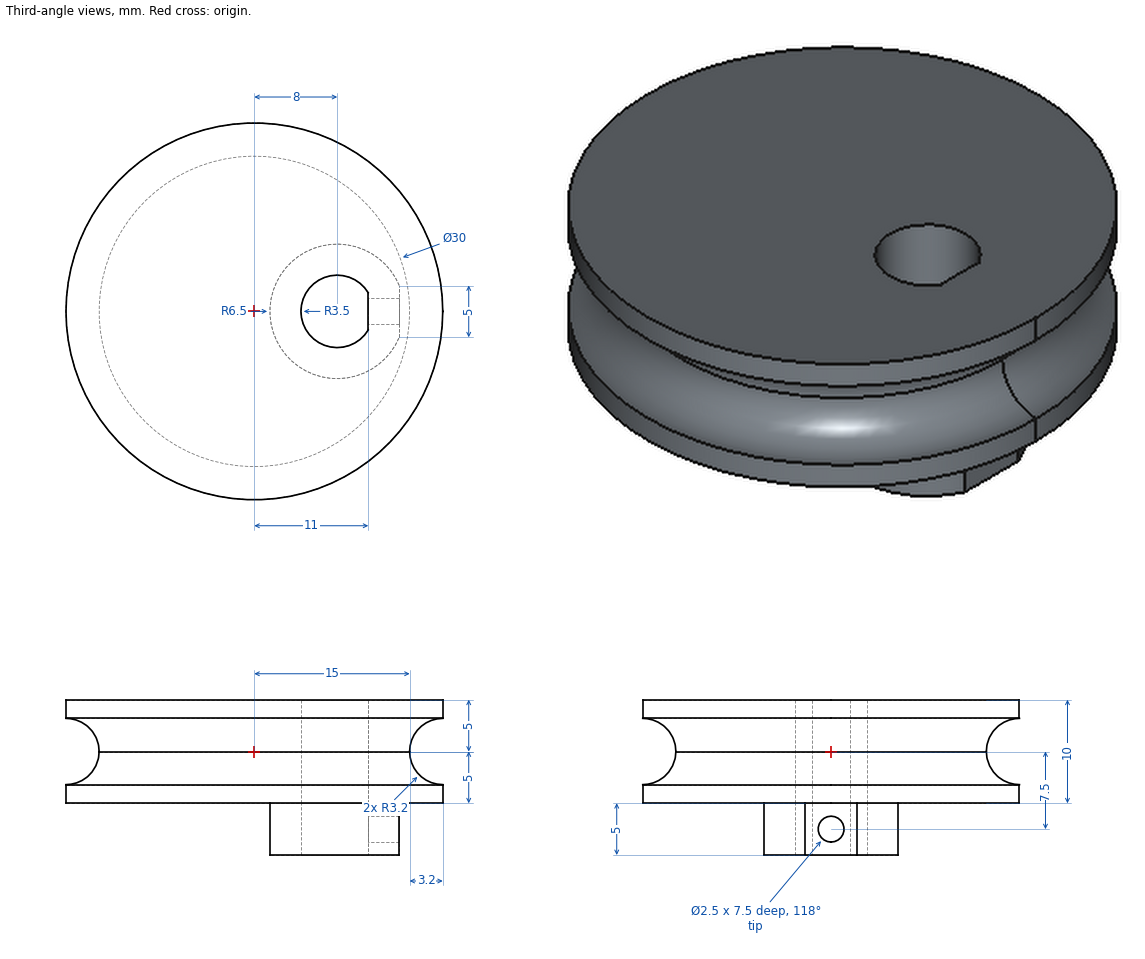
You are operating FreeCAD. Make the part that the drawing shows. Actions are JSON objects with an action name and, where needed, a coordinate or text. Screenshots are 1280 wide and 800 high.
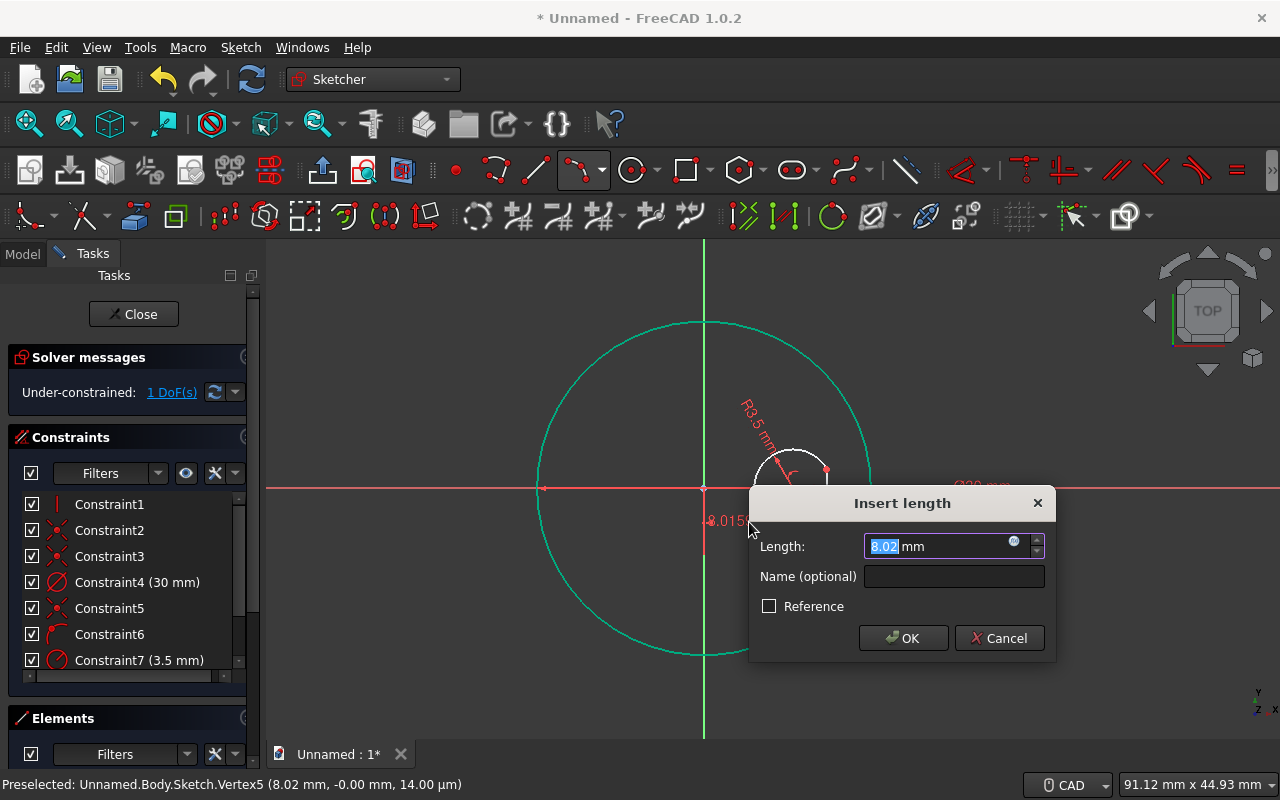
{"action": "type", "text": "8"}
{"action": "key", "text": "Return"}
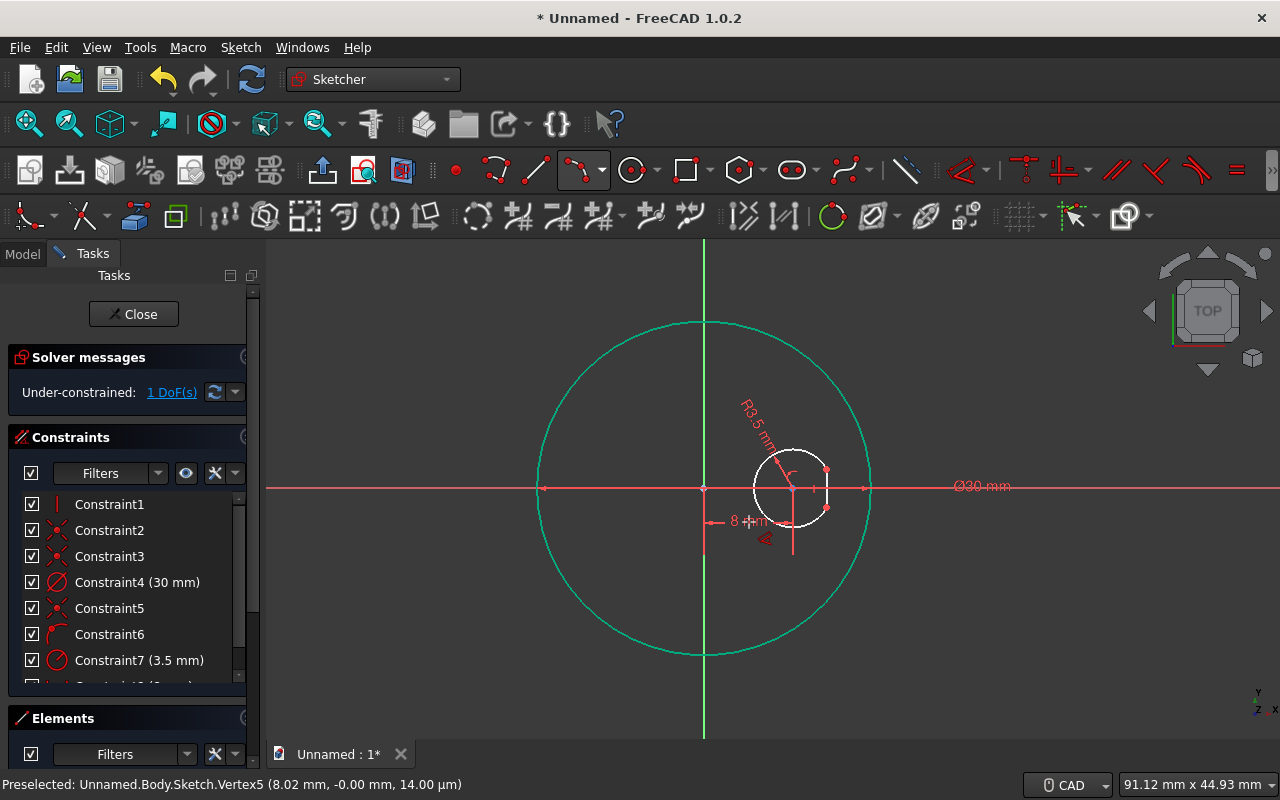
{"action": "left_click", "coordinate": [827, 508]}
{"action": "left_click", "coordinate": [737, 454]}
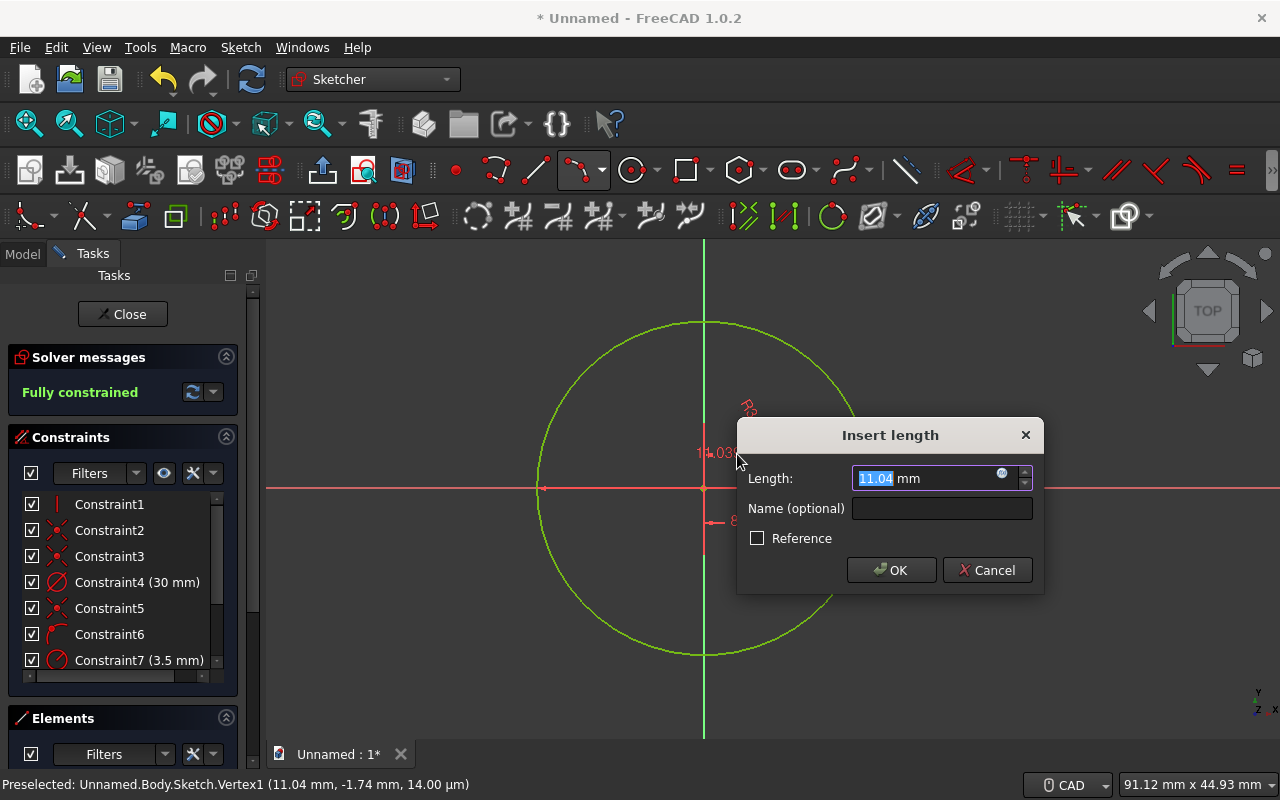
{"action": "type", "text": "11"}
{"action": "key", "text": "Return"}
{"action": "key", "text": "Escape"}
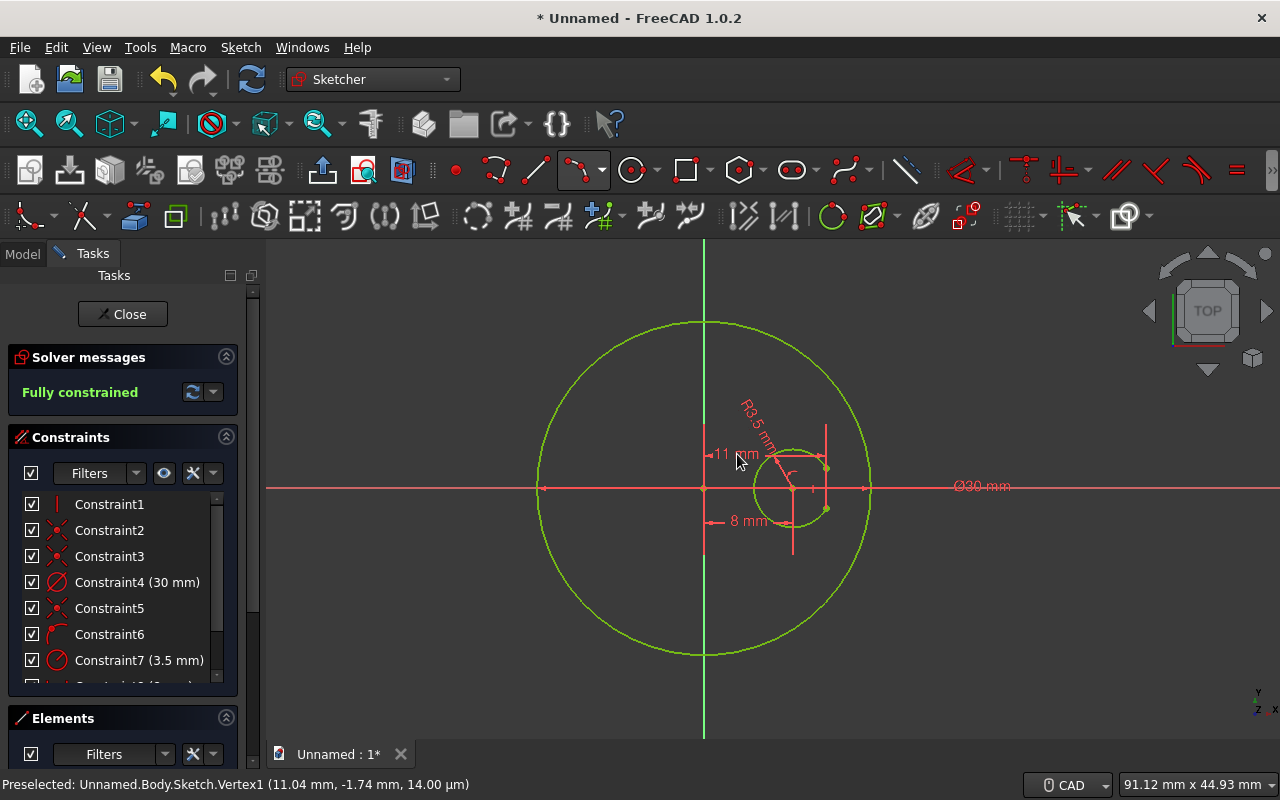
{"action": "left_click", "coordinate": [123, 314]}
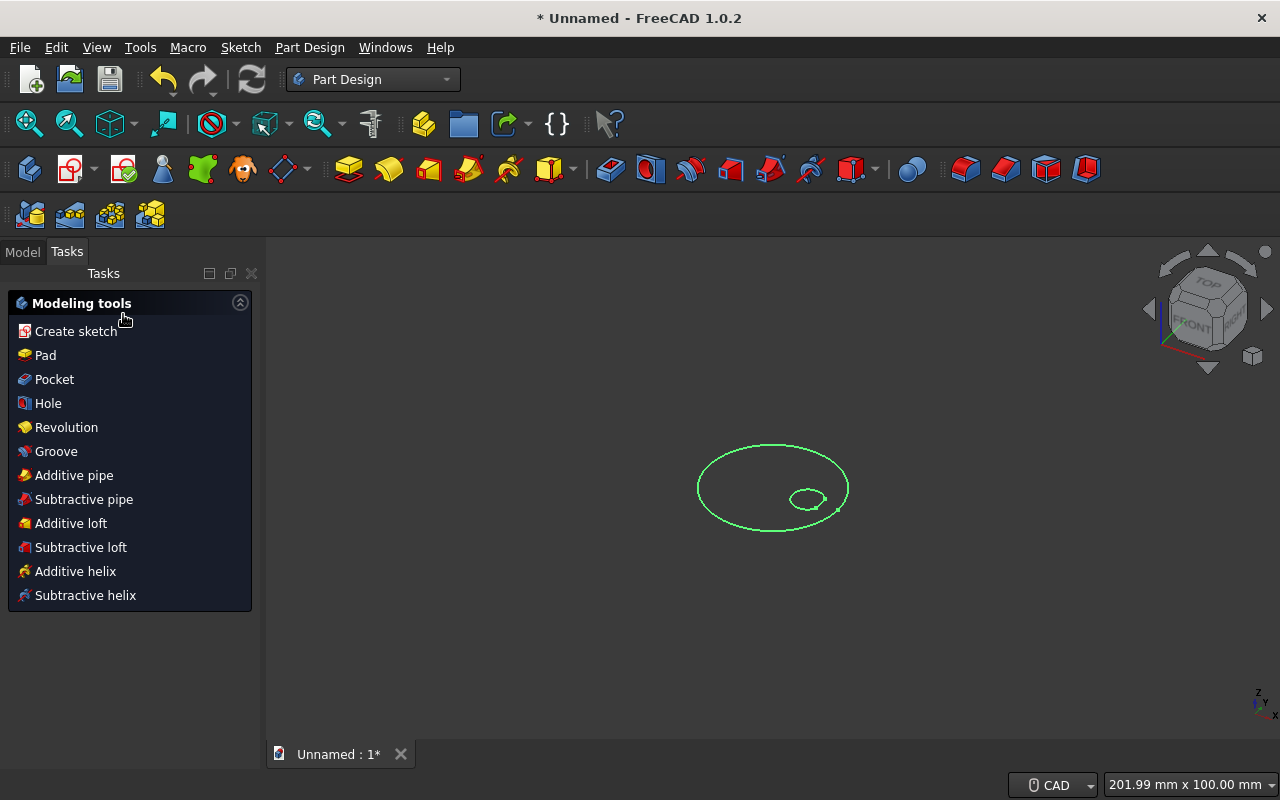
{"action": "left_click", "coordinate": [350, 170]}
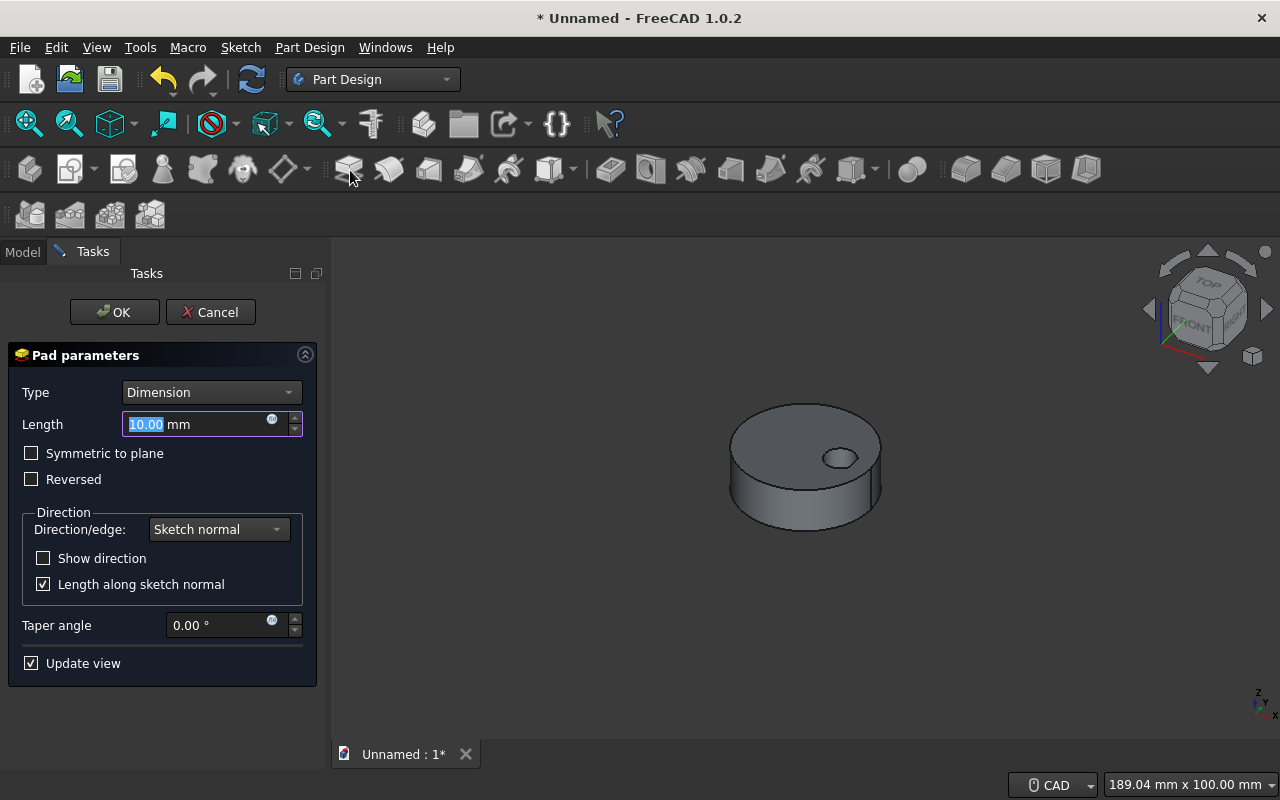
{"action": "type", "text": "10"}
{"action": "key", "text": "Tab"}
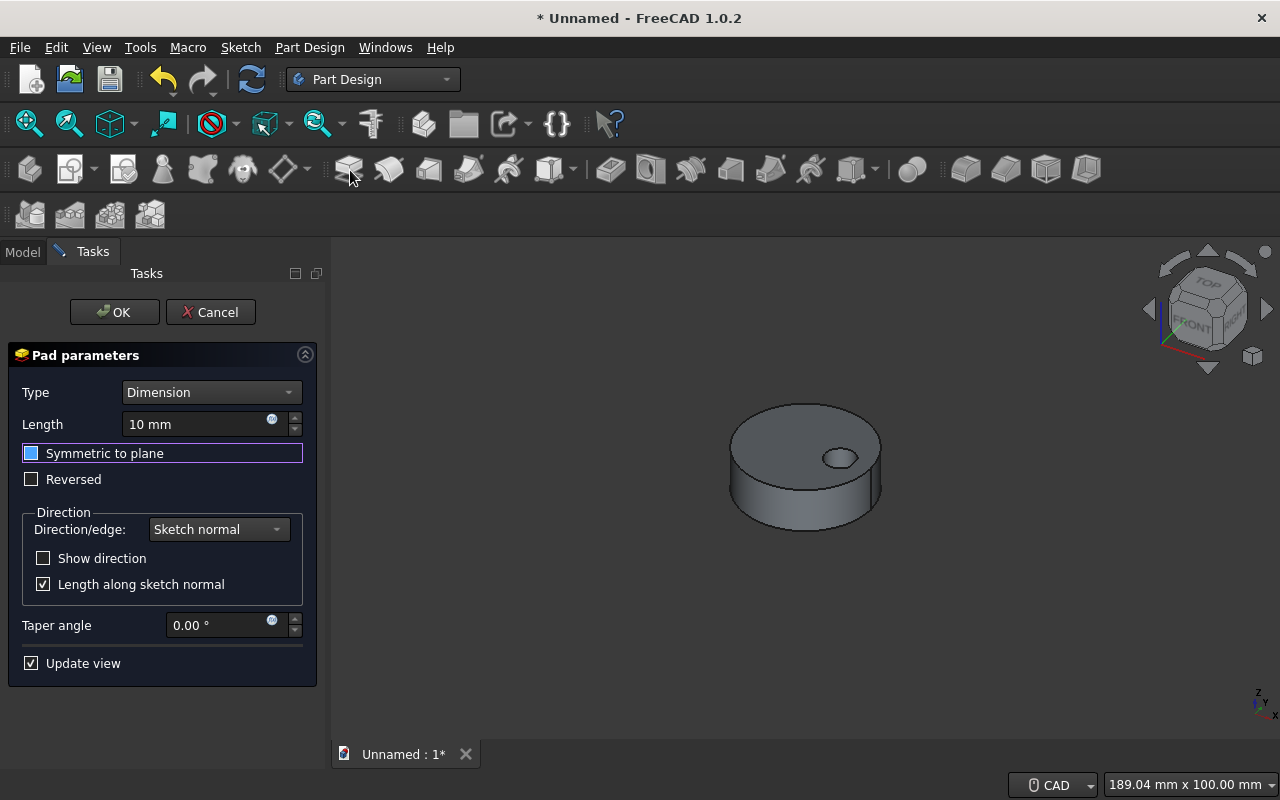
{"action": "left_click", "coordinate": [30, 453]}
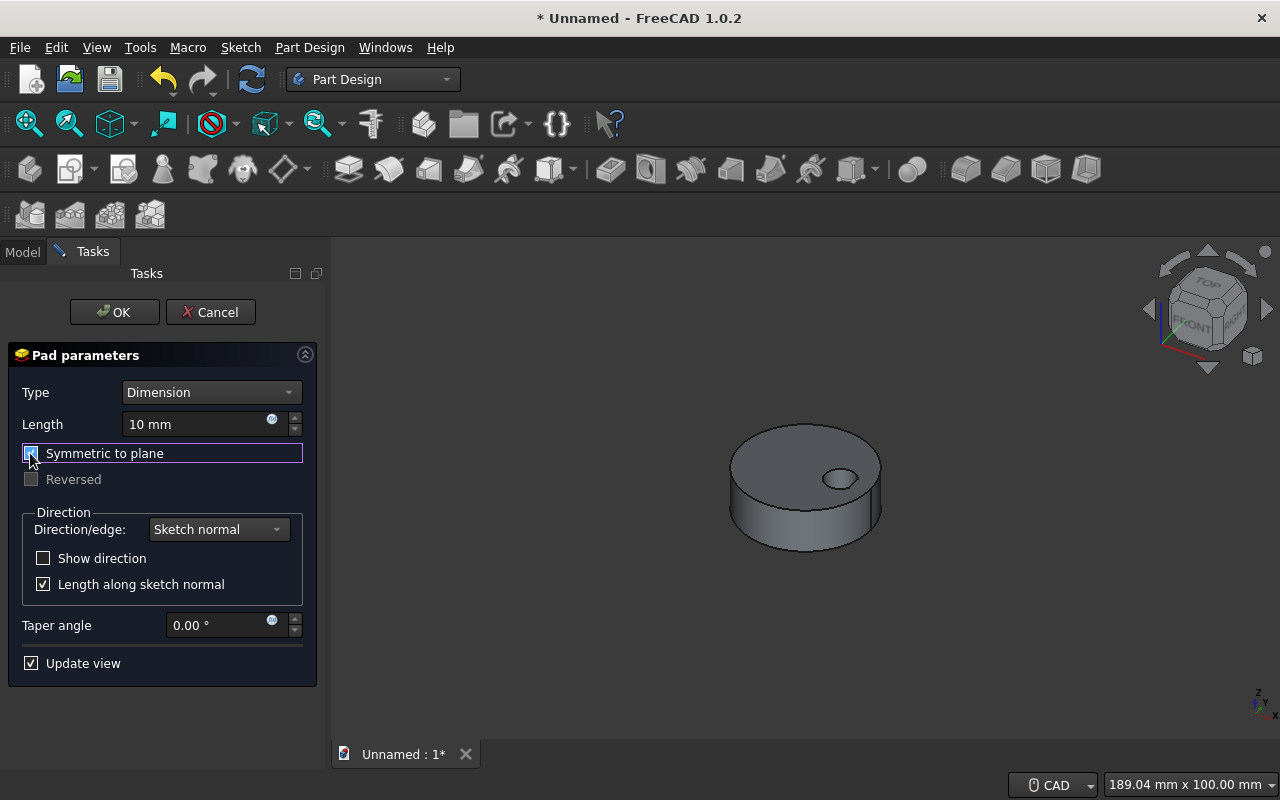
{"action": "left_click", "coordinate": [115, 312]}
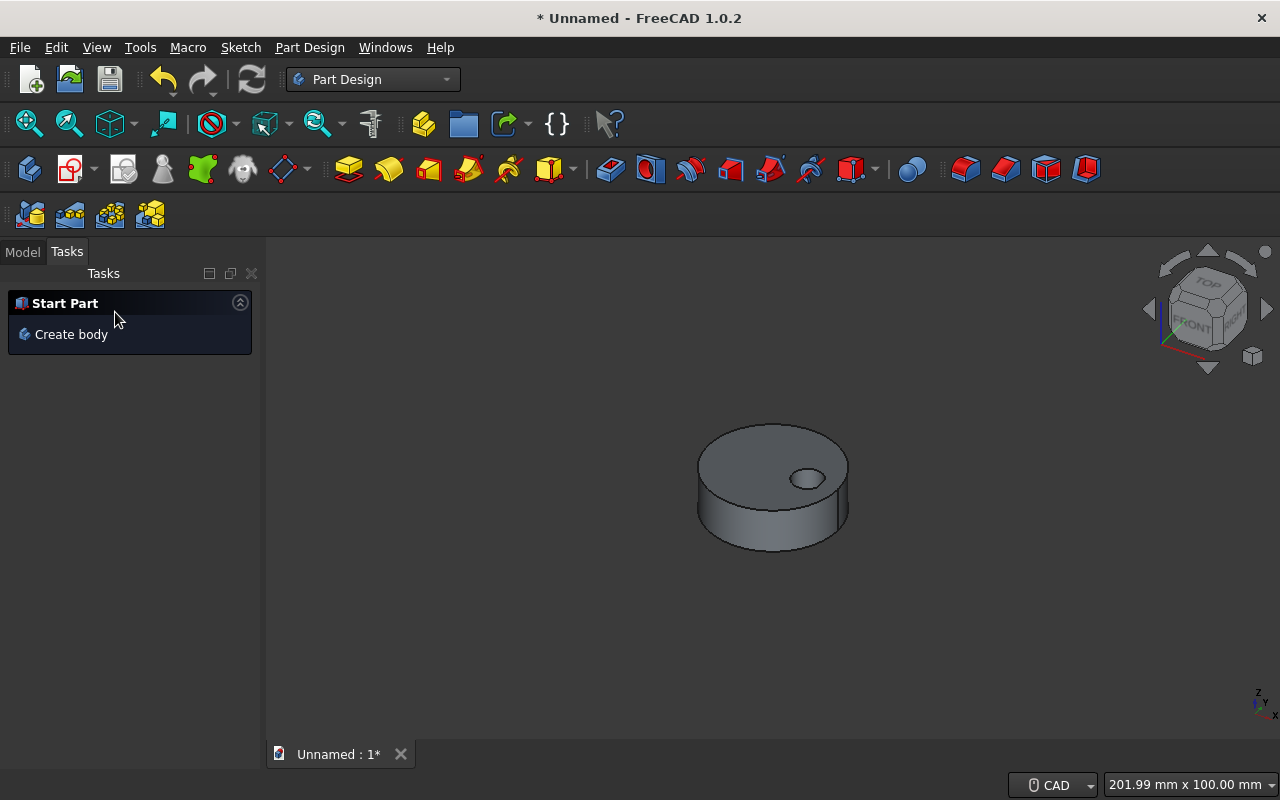
{"action": "left_click", "coordinate": [30, 124]}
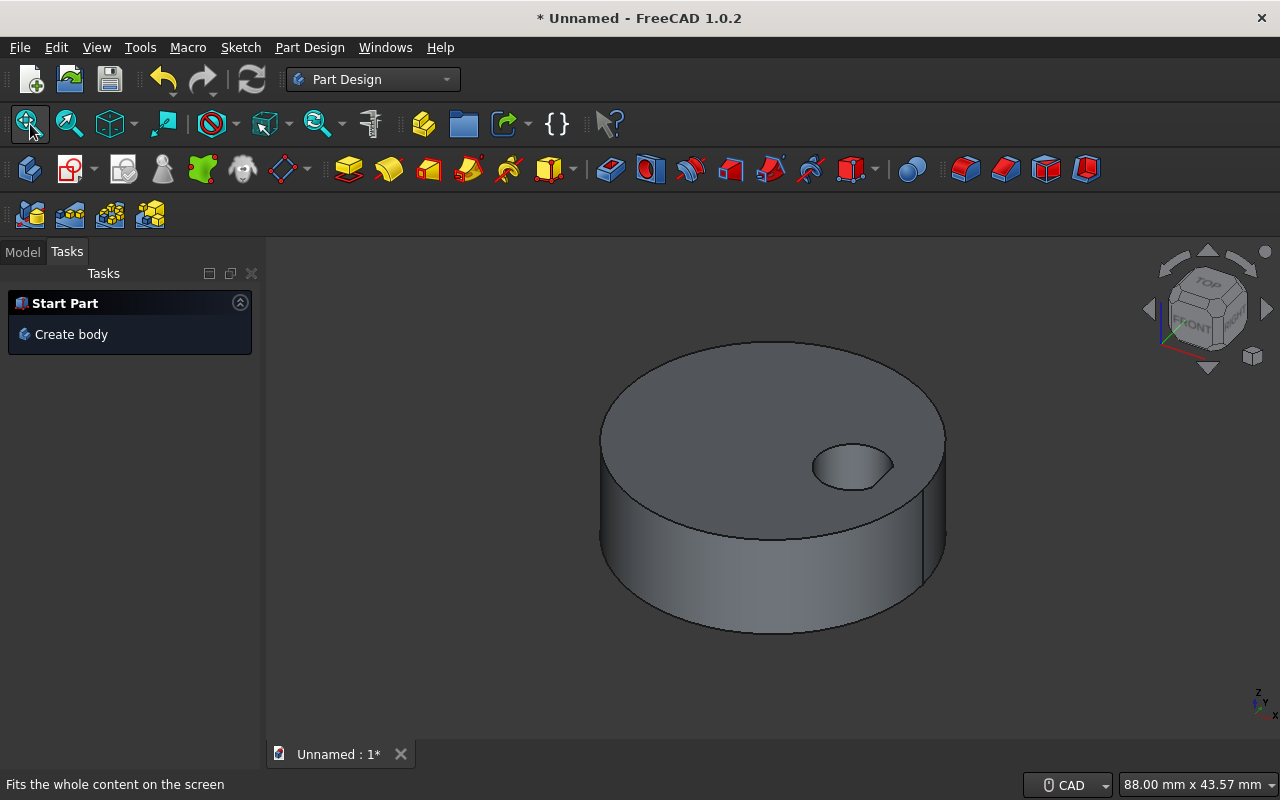
{"action": "left_click", "coordinate": [70, 170]}